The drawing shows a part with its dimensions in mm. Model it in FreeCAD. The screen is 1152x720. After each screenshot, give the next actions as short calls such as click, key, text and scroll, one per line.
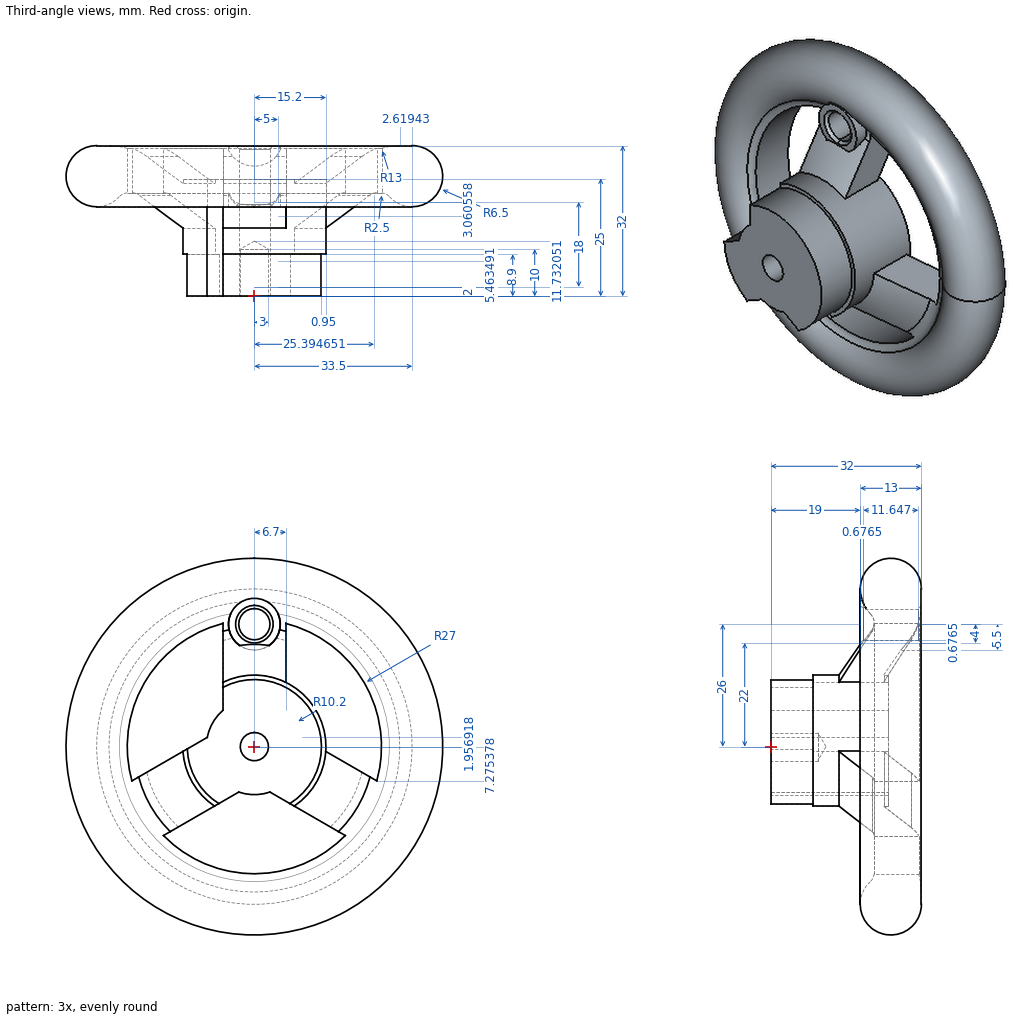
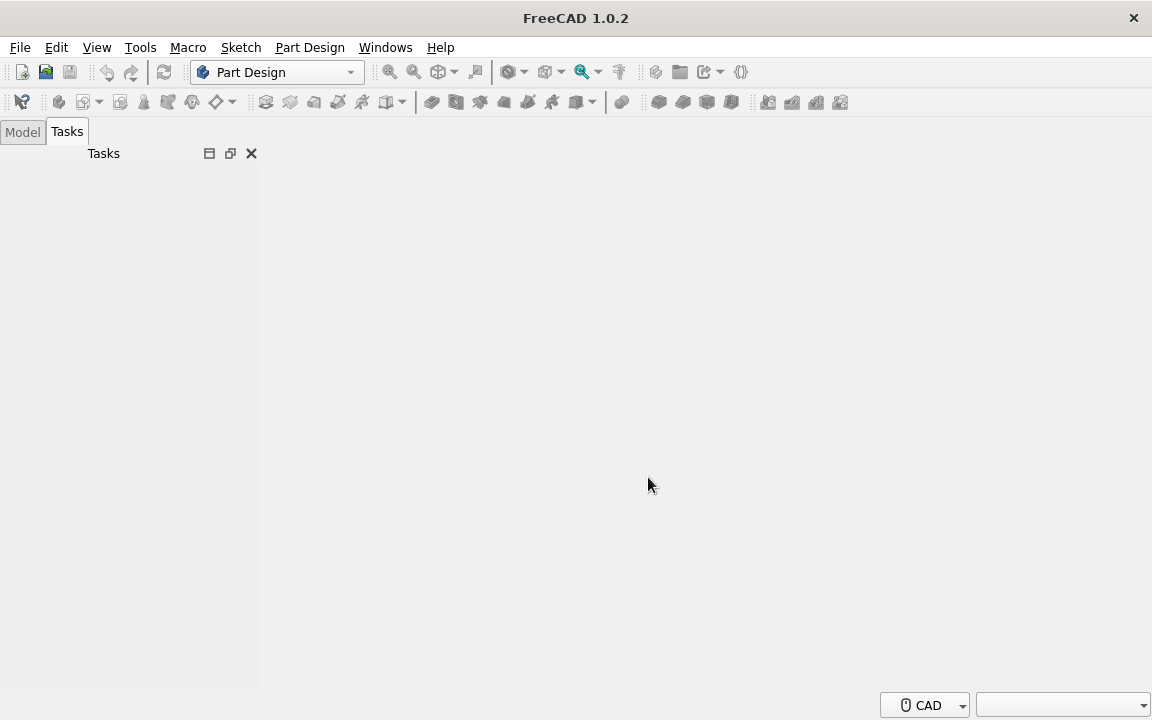
click(22, 72)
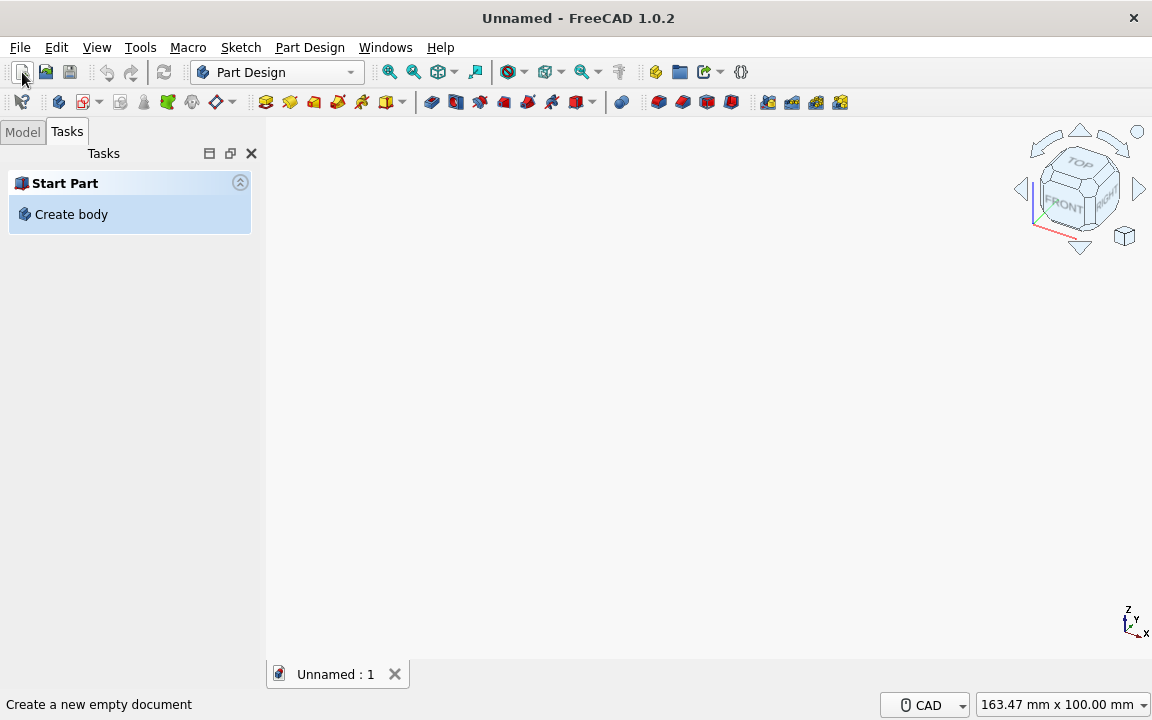
click(84, 102)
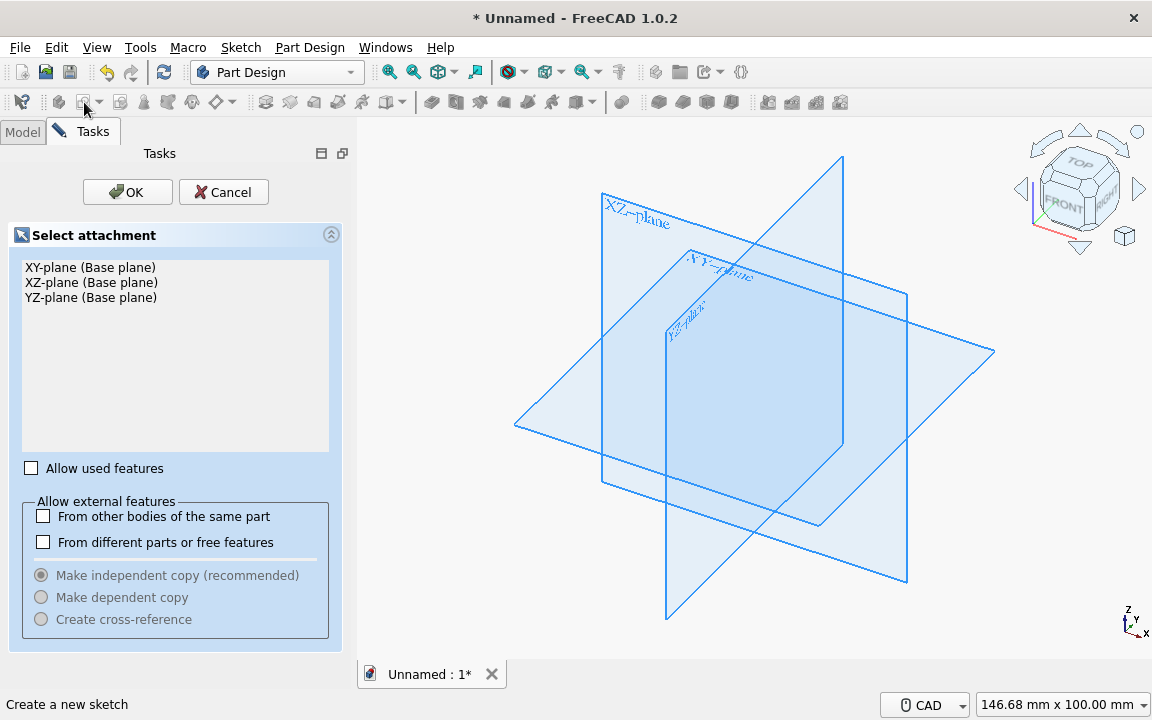
click(82, 268)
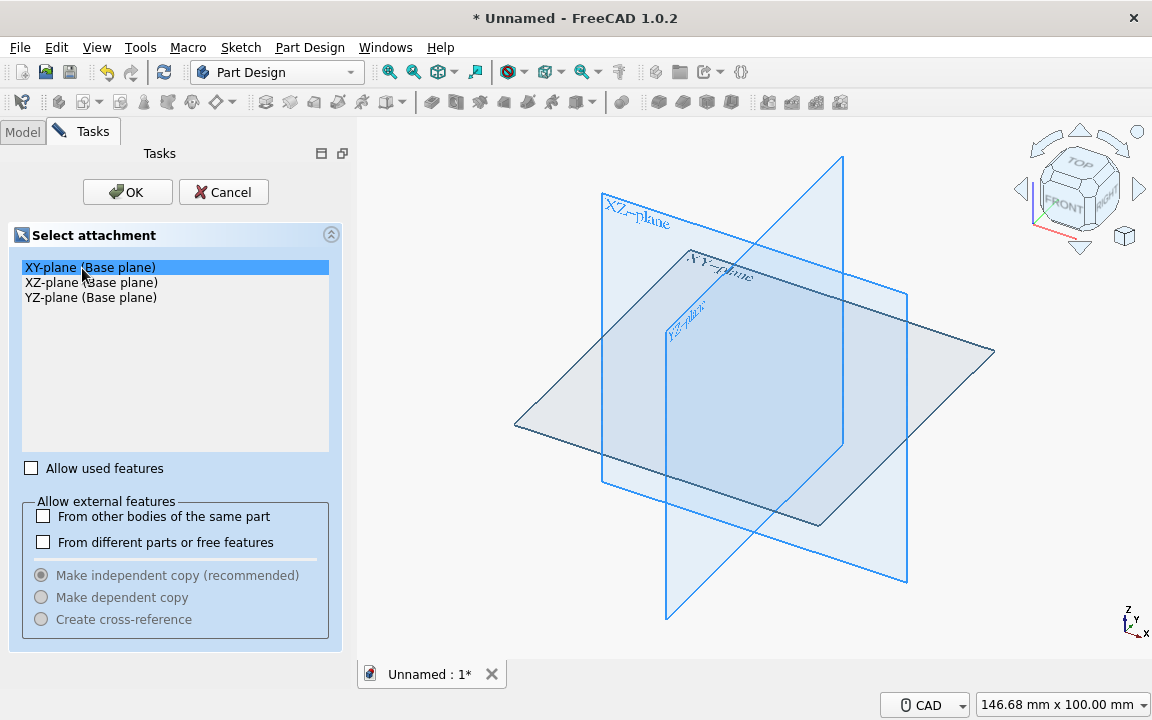
click(128, 192)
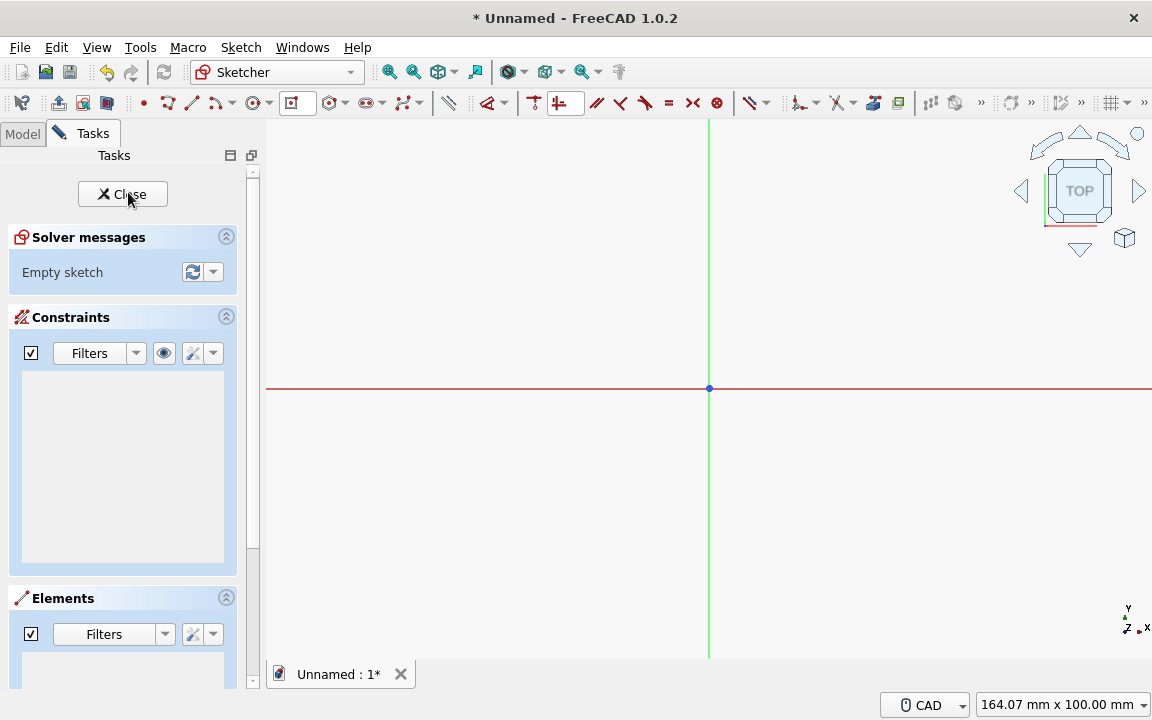
scroll(987, 198, up, 3)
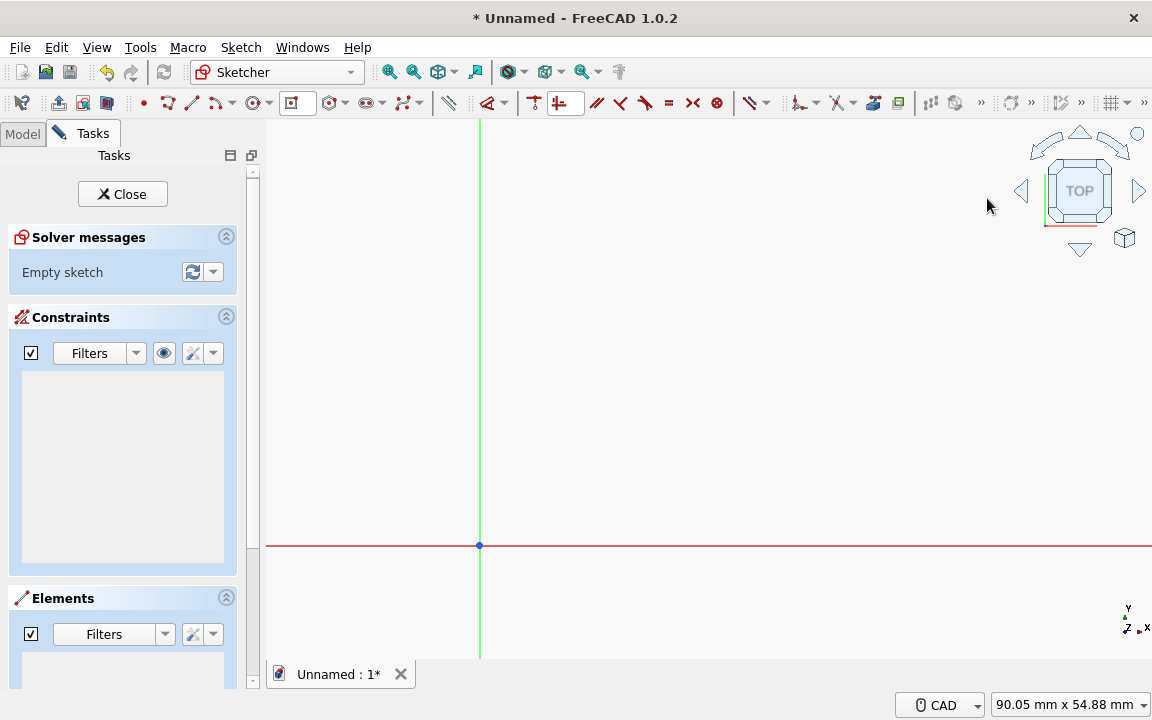
key(g)
key(l)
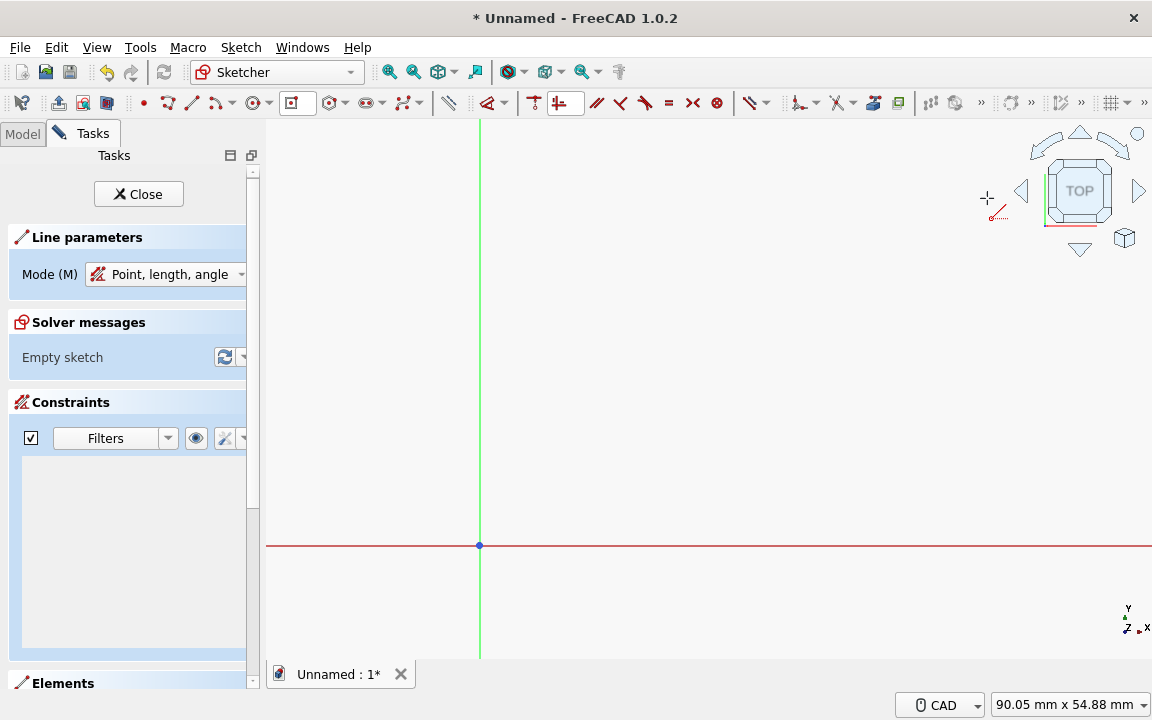
click(809, 231)
click(784, 231)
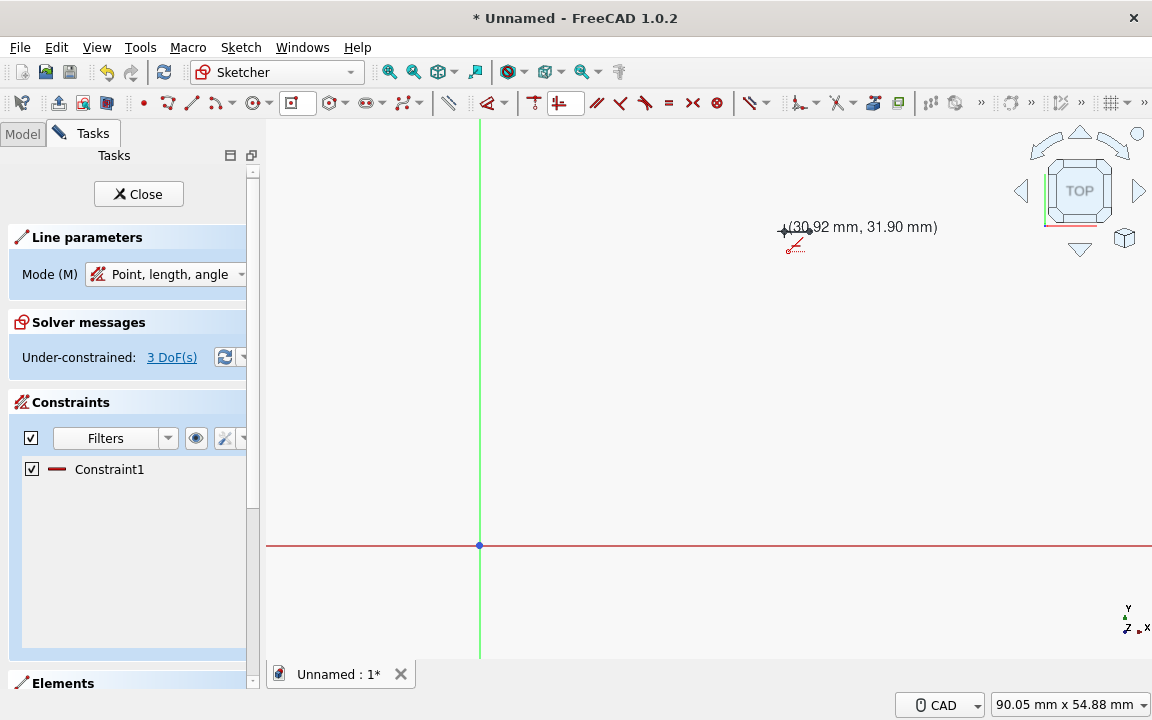
key(g)
key(m)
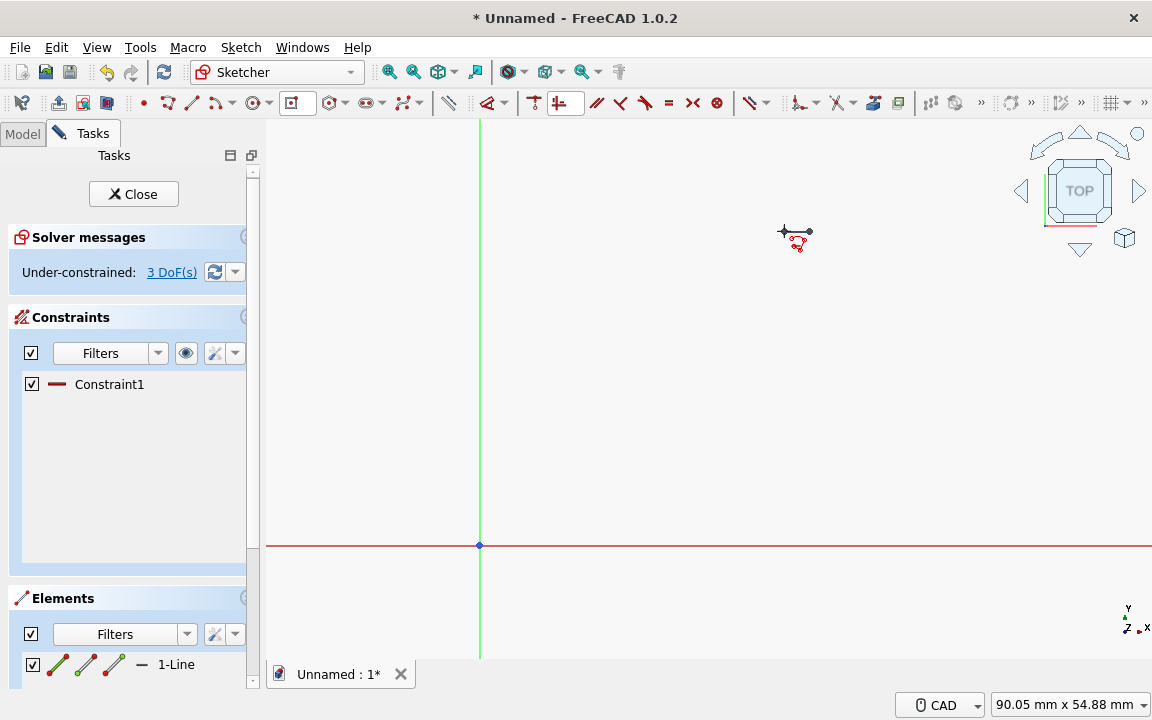
click(711, 254)
click(529, 379)
click(529, 349)
click(480, 349)
click(489, 526)
click(529, 526)
click(529, 472)
click(730, 334)
right_click(730, 334)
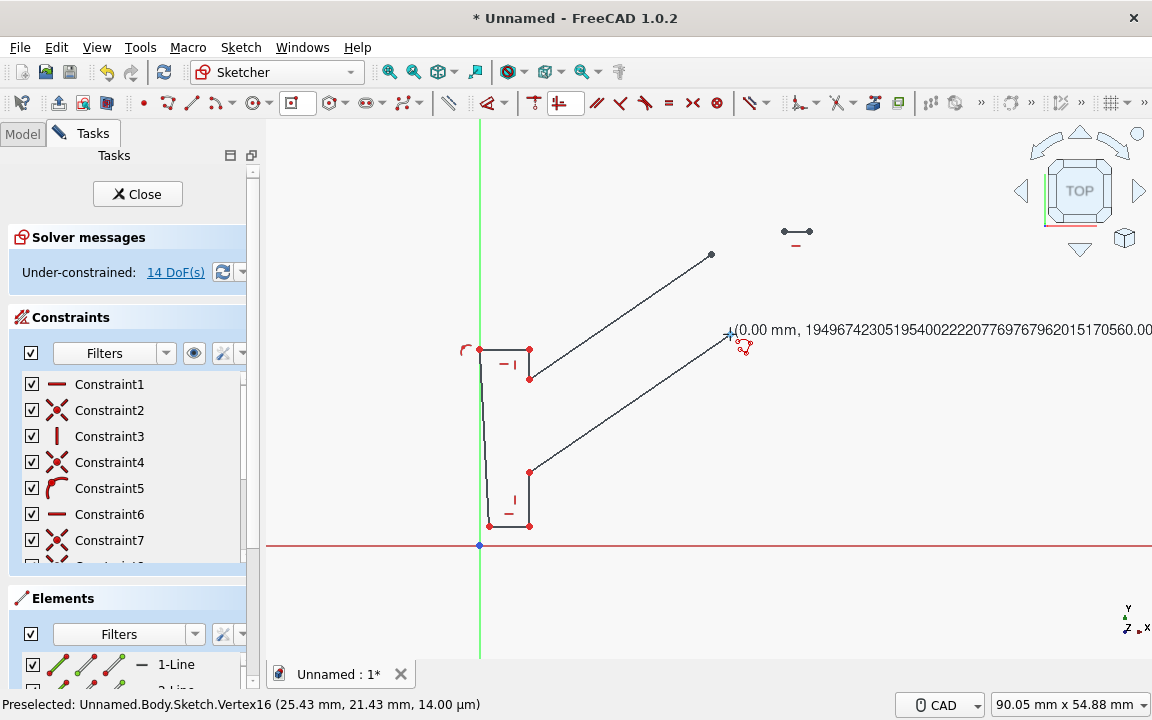
key(g)
key(3)
key(a)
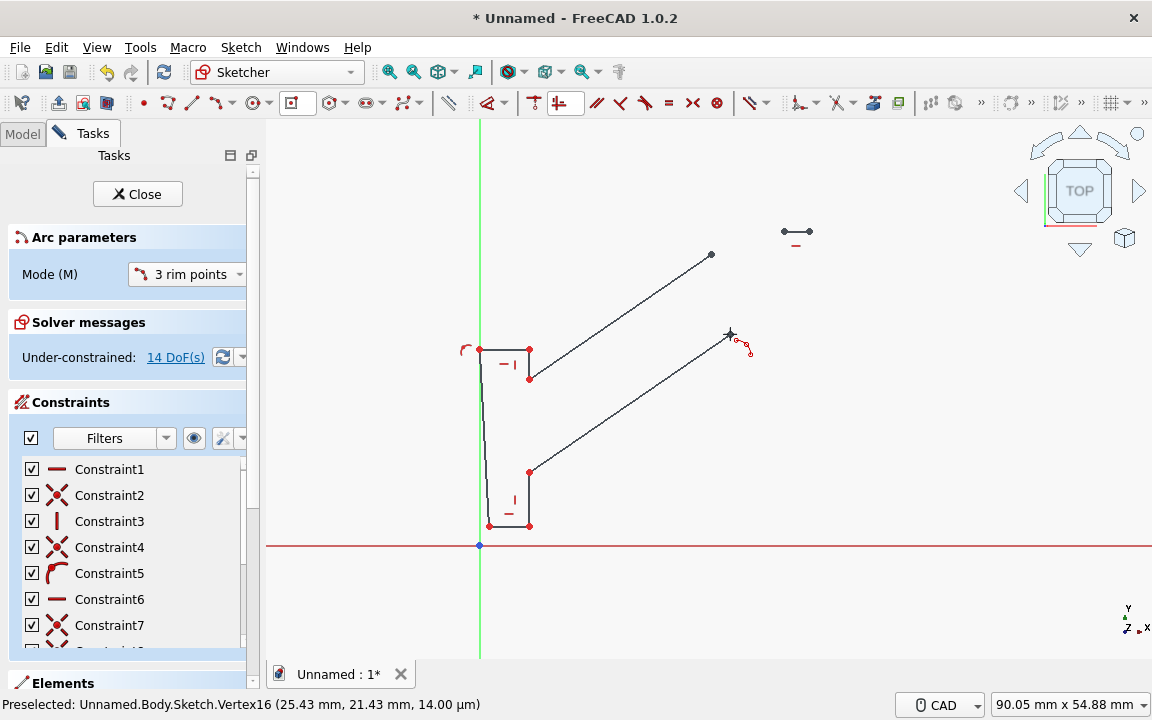
scroll(784, 231, up, 2)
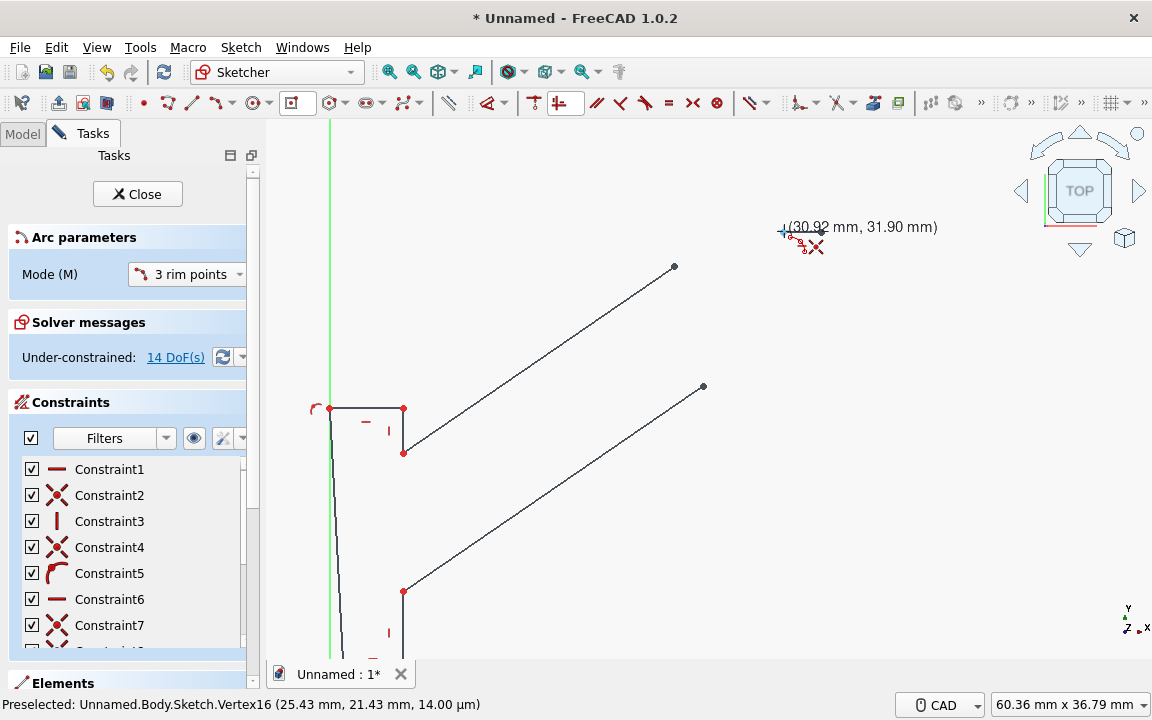
click(784, 232)
click(675, 267)